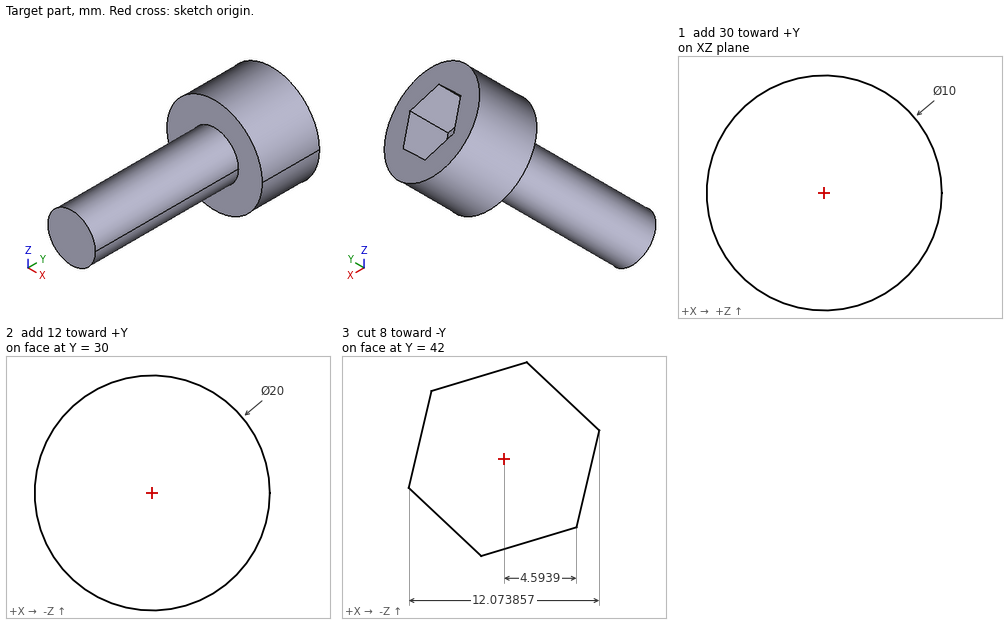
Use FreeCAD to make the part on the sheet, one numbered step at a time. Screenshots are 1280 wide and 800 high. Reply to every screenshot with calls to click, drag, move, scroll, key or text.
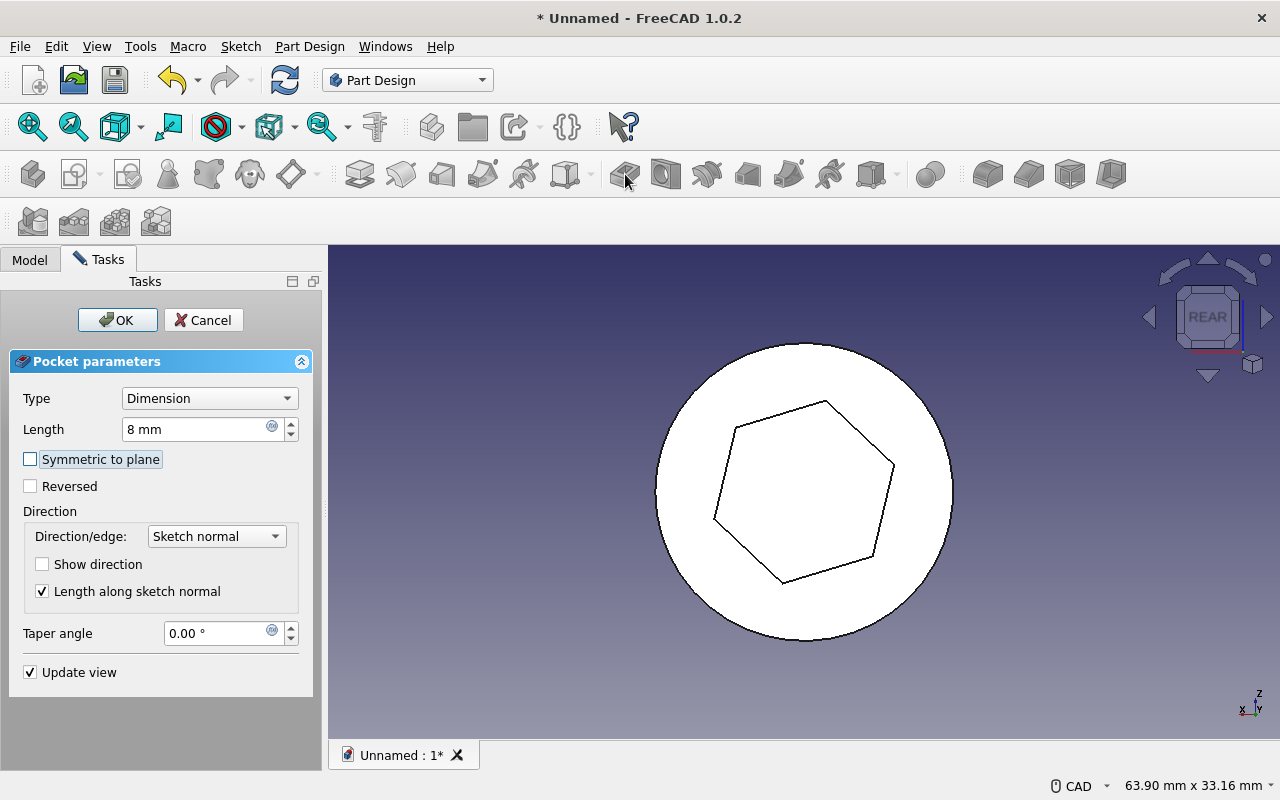
click(118, 320)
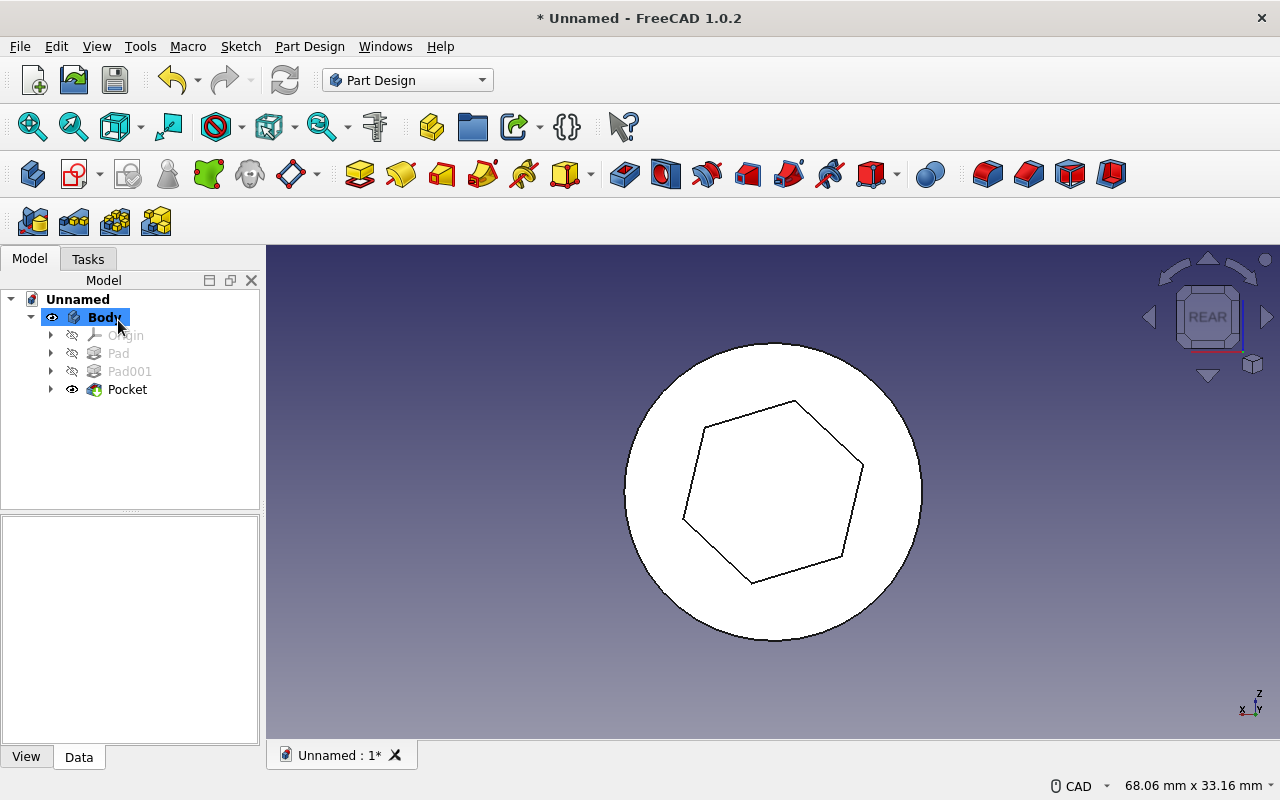
key(0)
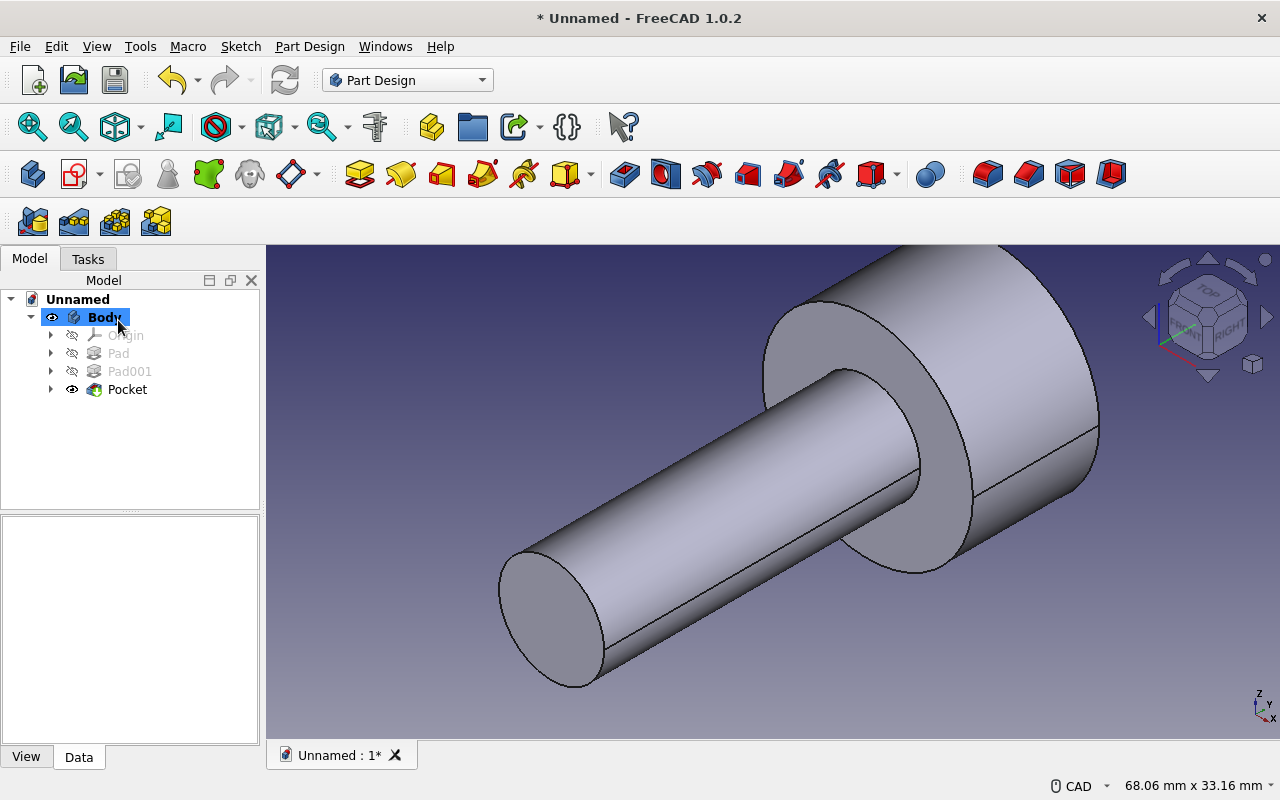
click(33, 128)